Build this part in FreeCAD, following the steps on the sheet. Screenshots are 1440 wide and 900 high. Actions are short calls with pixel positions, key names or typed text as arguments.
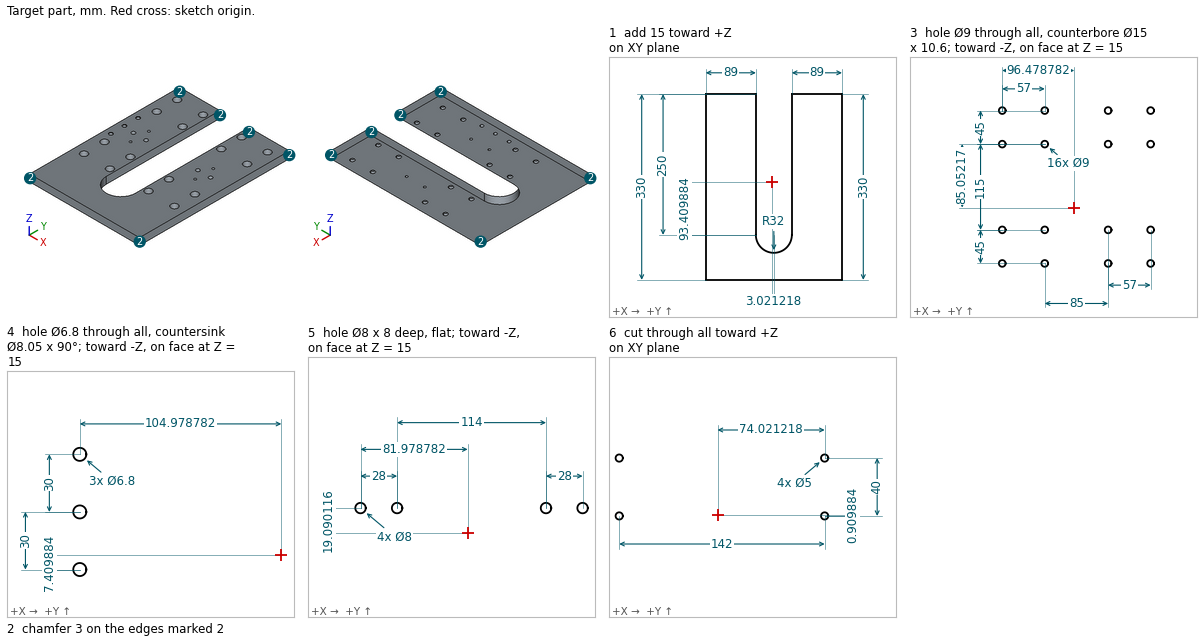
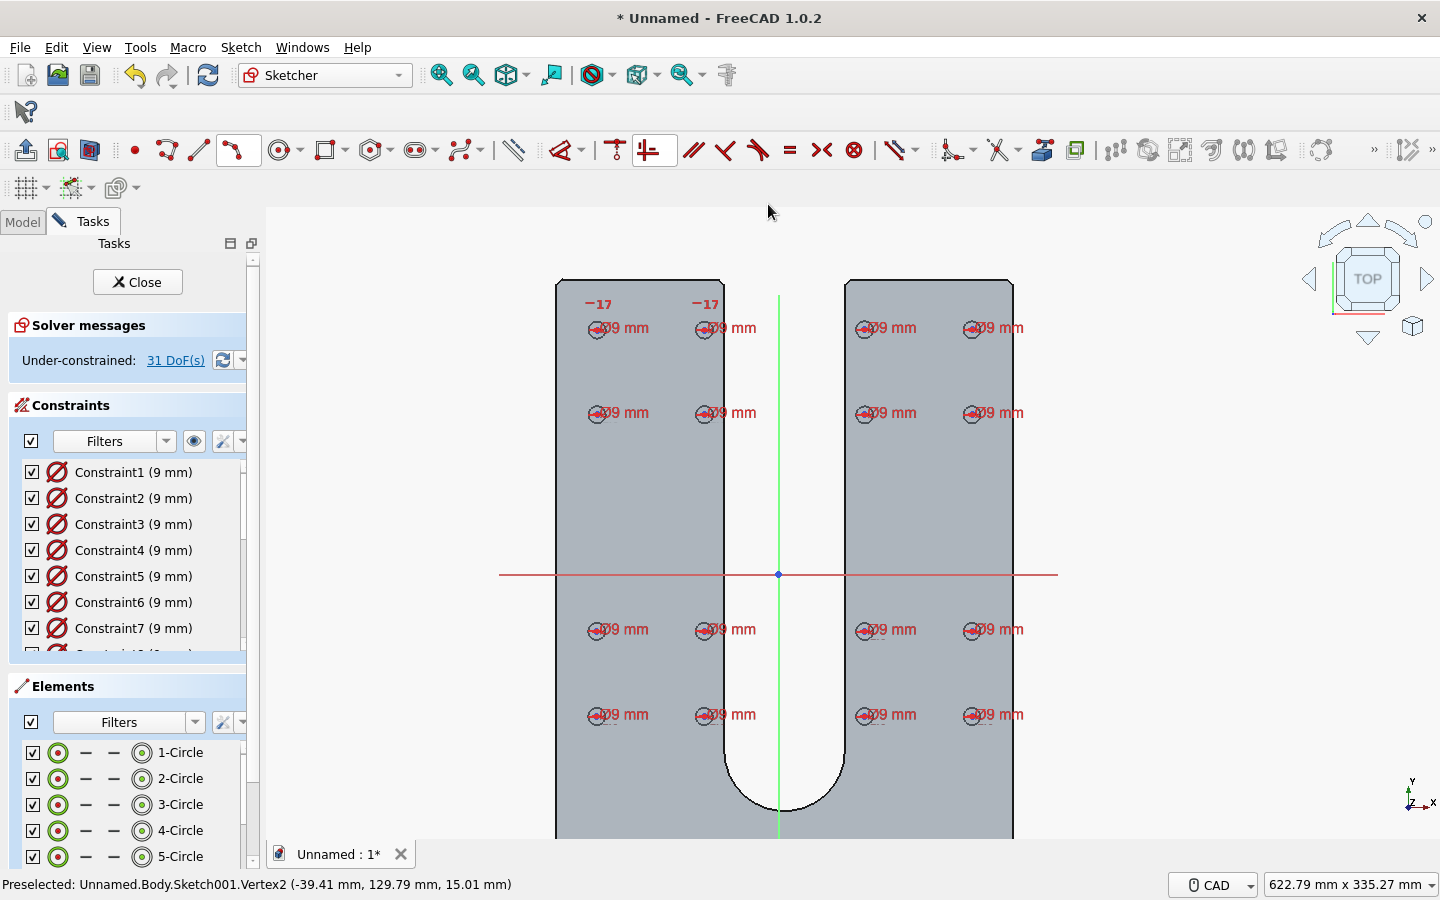
click(705, 330)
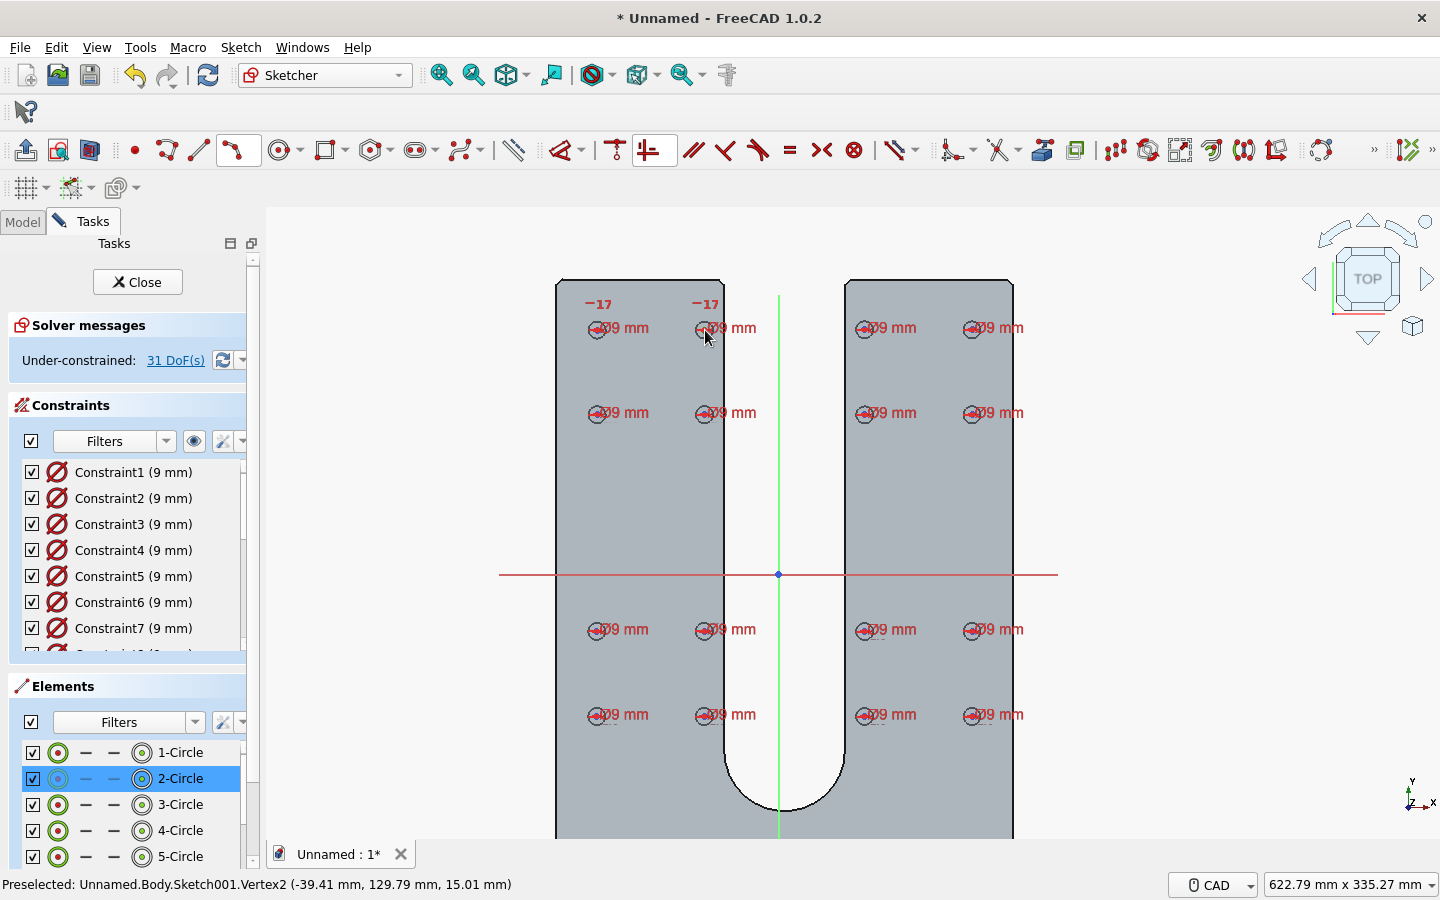
click(705, 415)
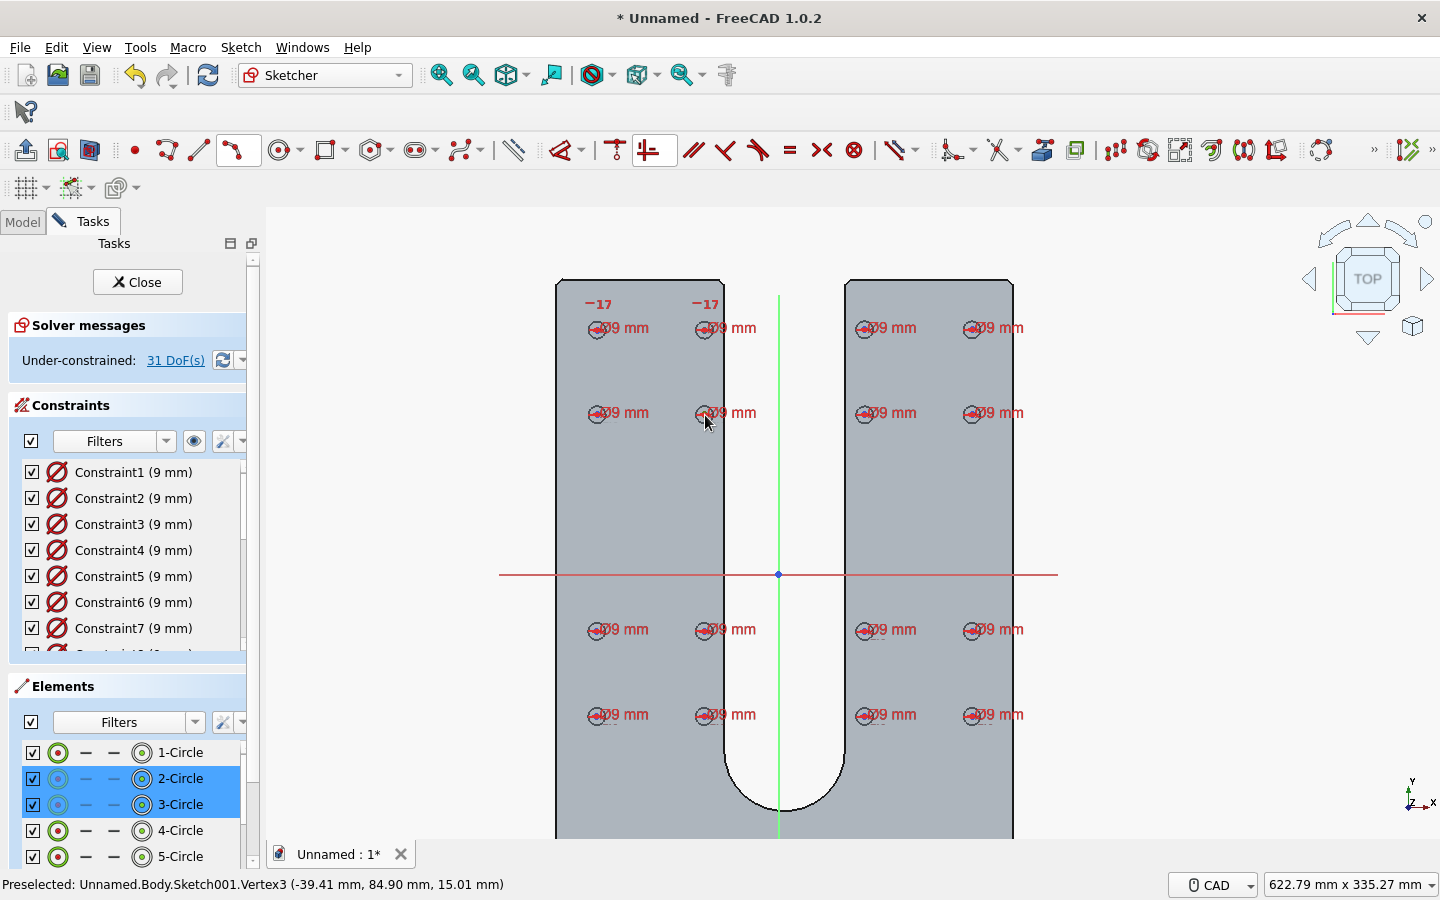
key(v)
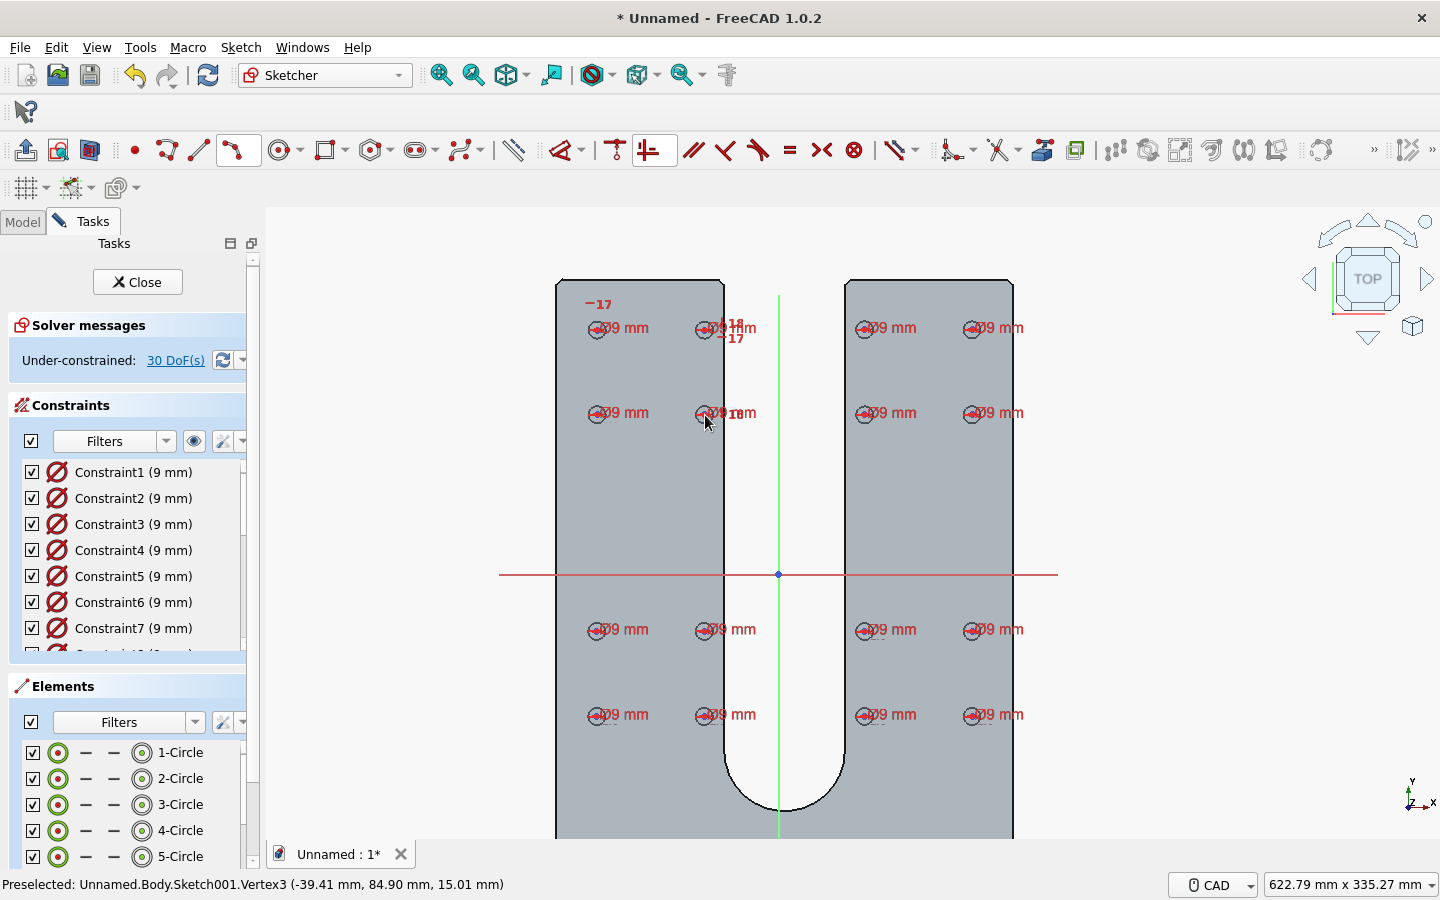
click(597, 330)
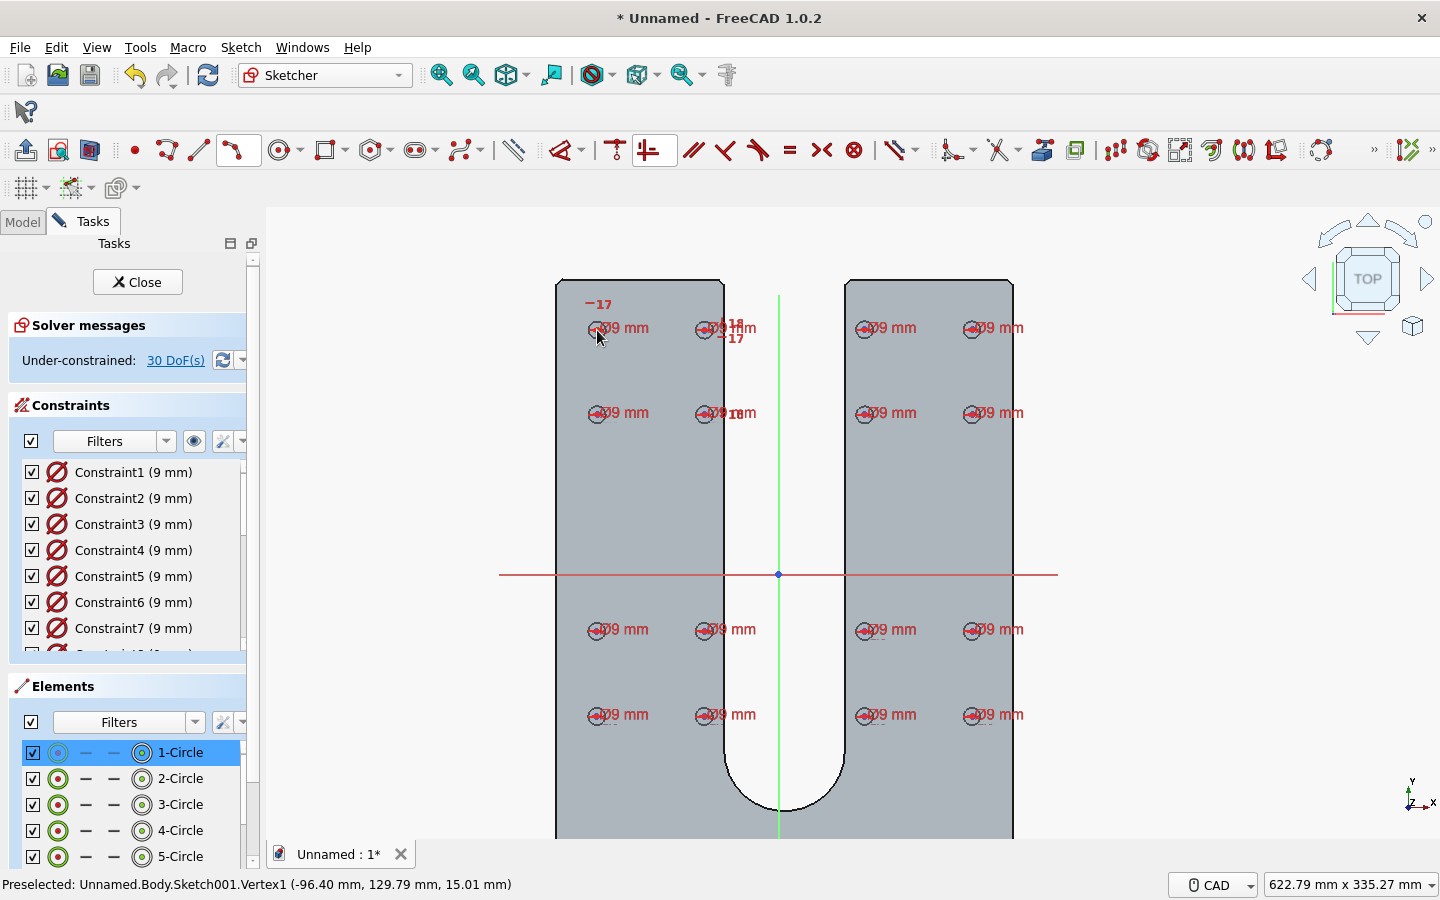
click(597, 415)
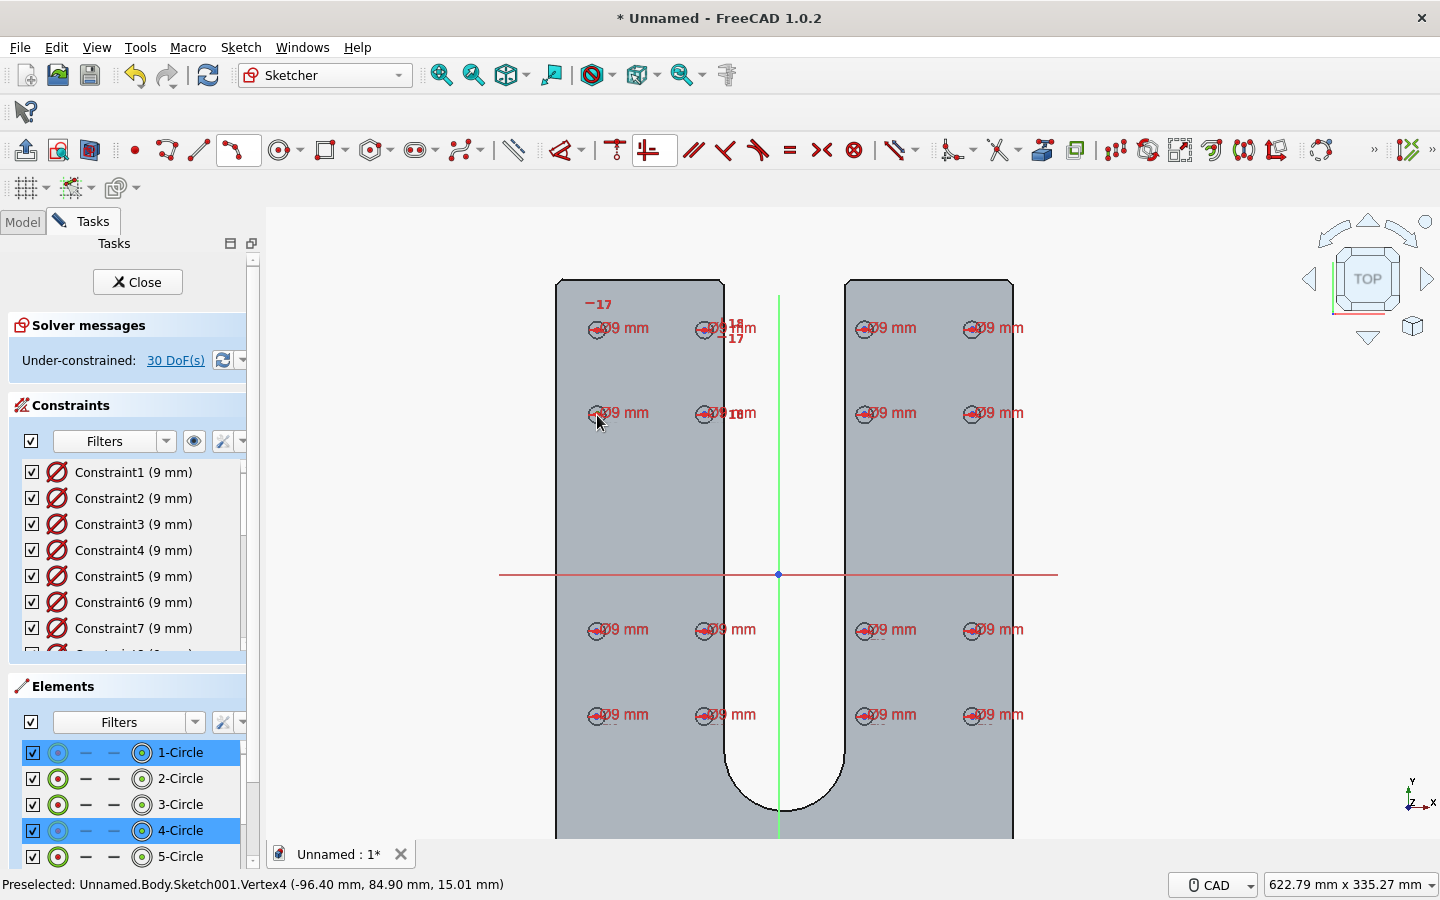
click(672, 150)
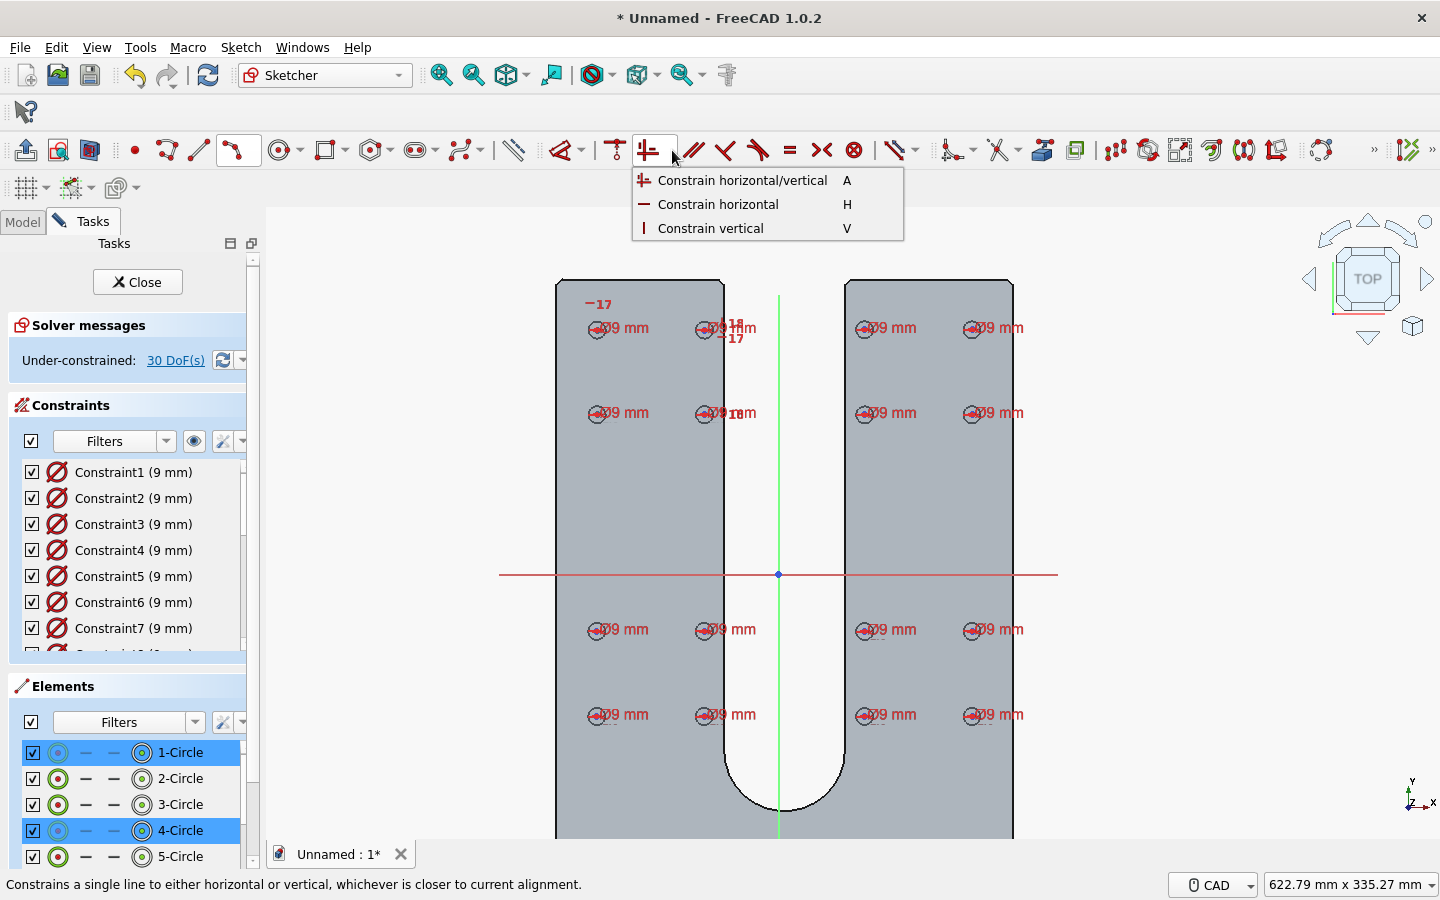
click(768, 228)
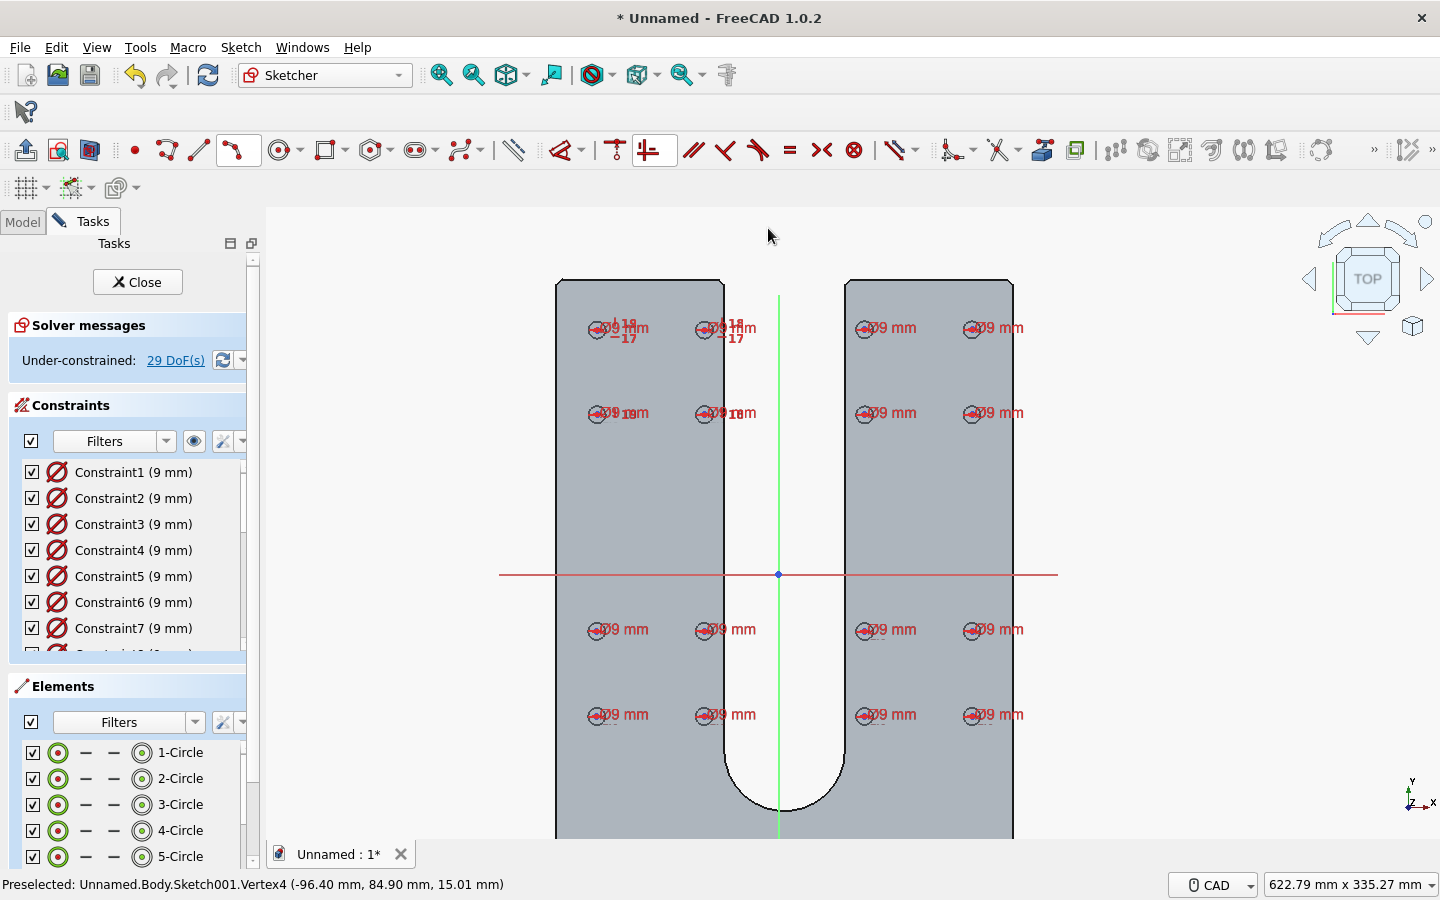
click(705, 415)